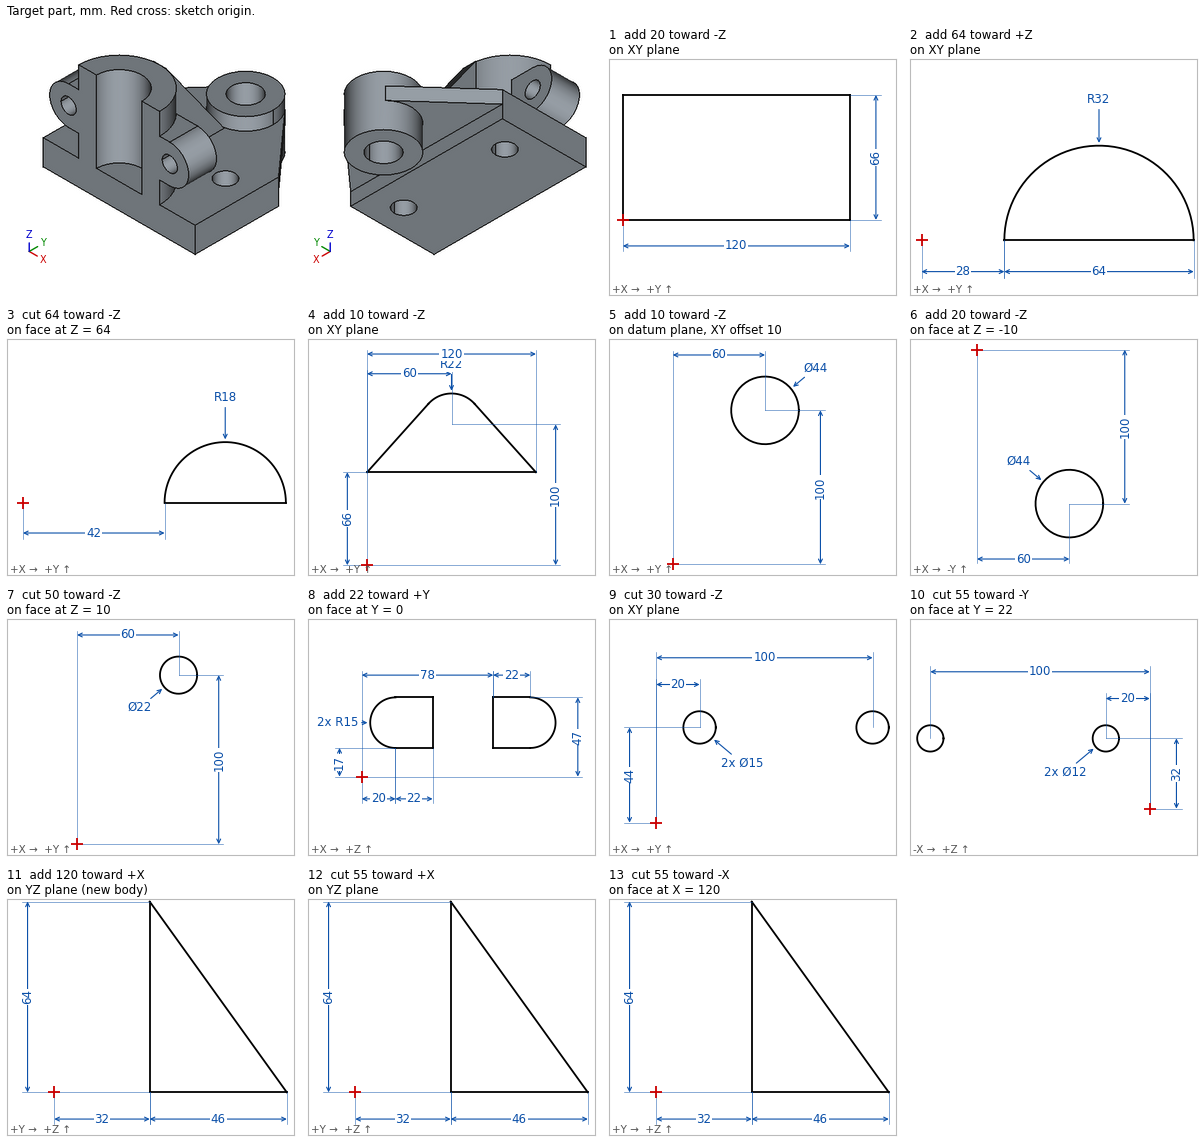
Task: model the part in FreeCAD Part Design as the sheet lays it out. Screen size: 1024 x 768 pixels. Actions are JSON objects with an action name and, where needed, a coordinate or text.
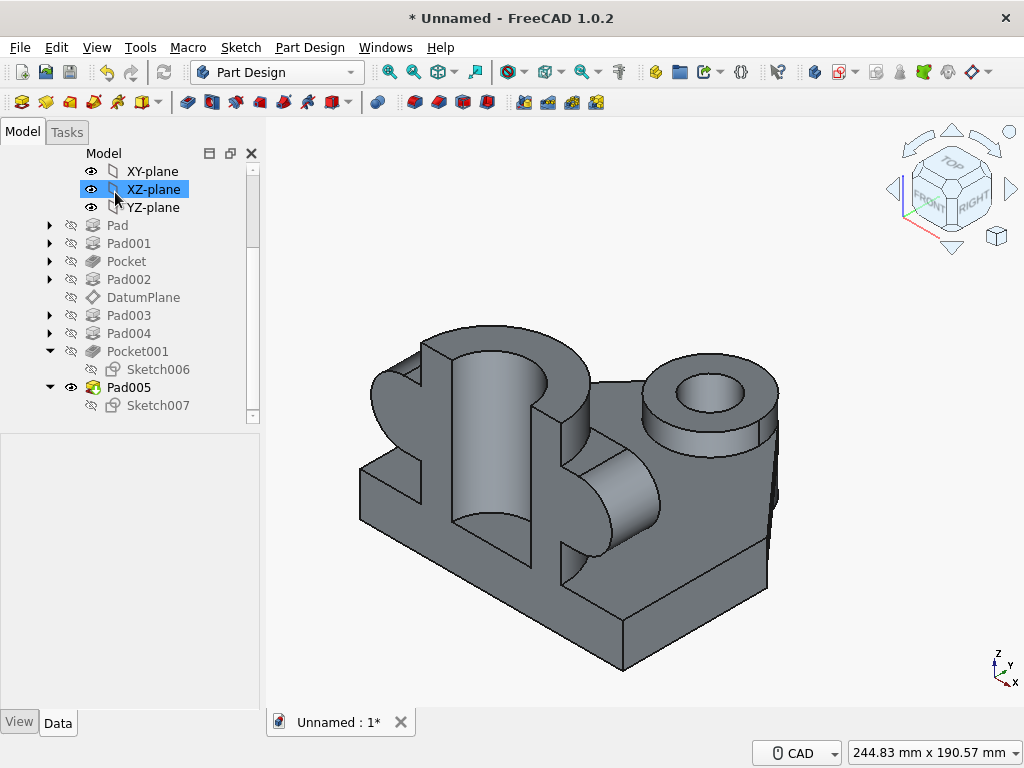
{"action": "left_click", "coordinate": [840, 72]}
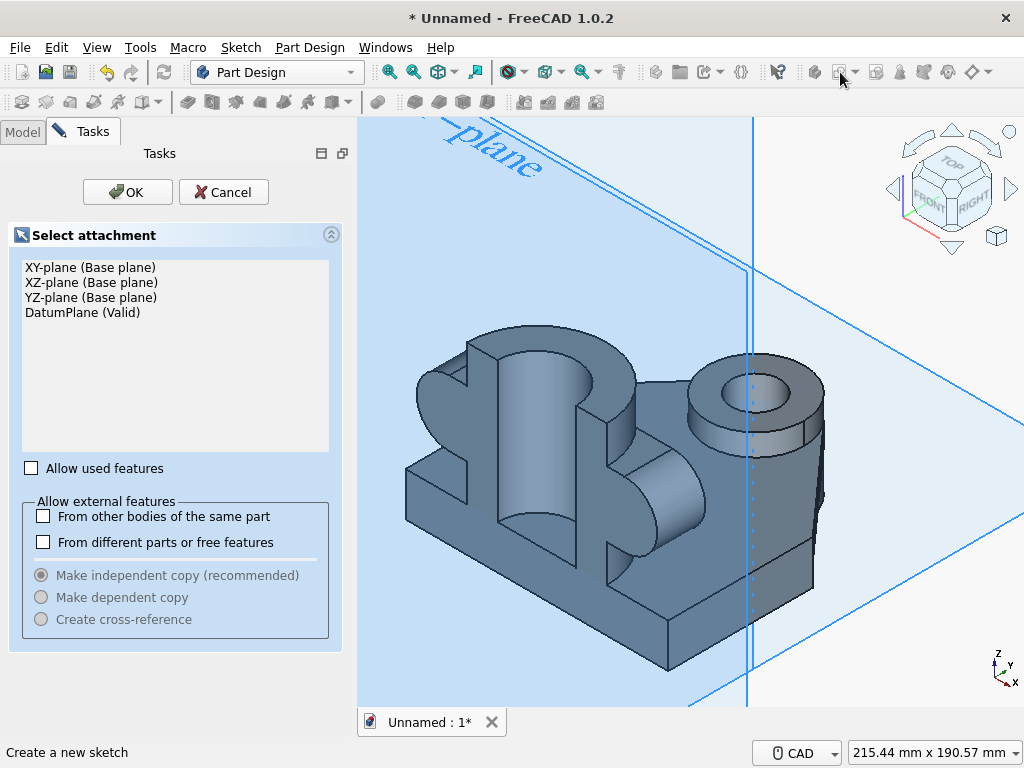
{"action": "left_click", "coordinate": [82, 268]}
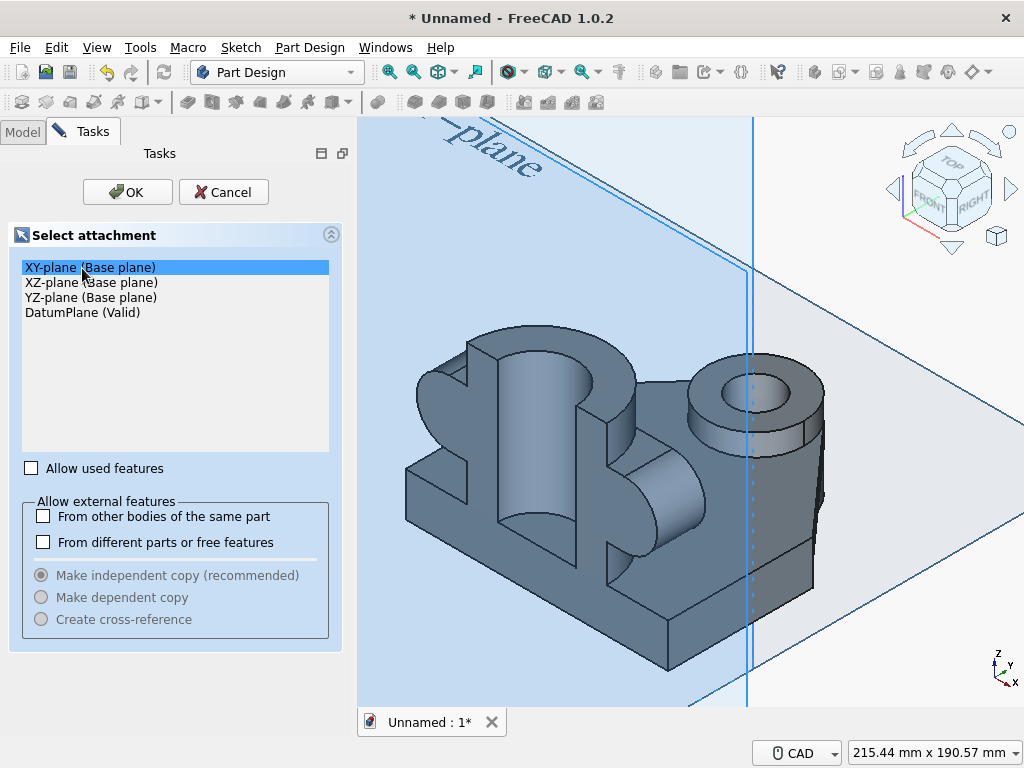
{"action": "left_click", "coordinate": [128, 192]}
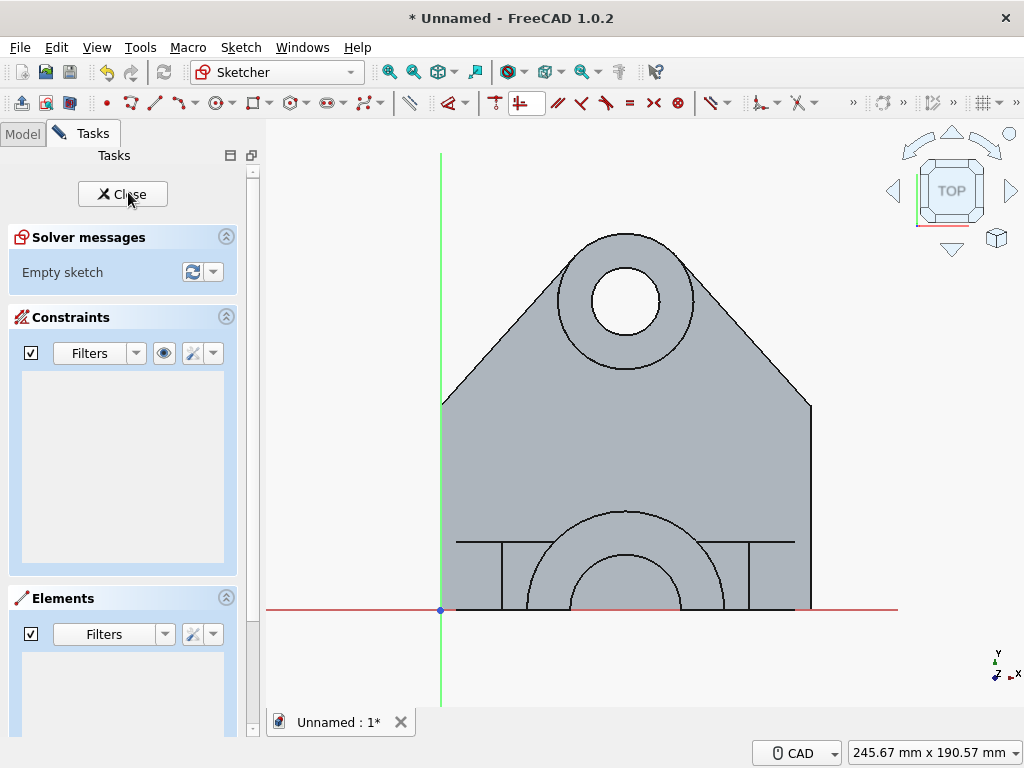
{"action": "left_click", "coordinate": [70, 104]}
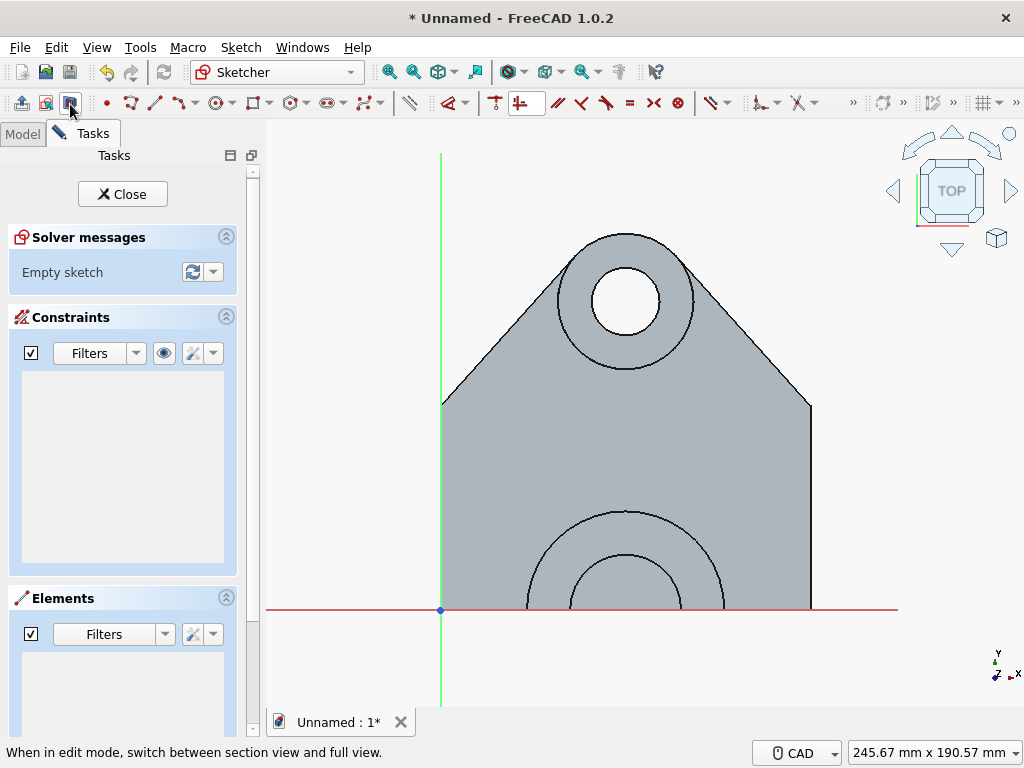
{"action": "left_click", "coordinate": [216, 104]}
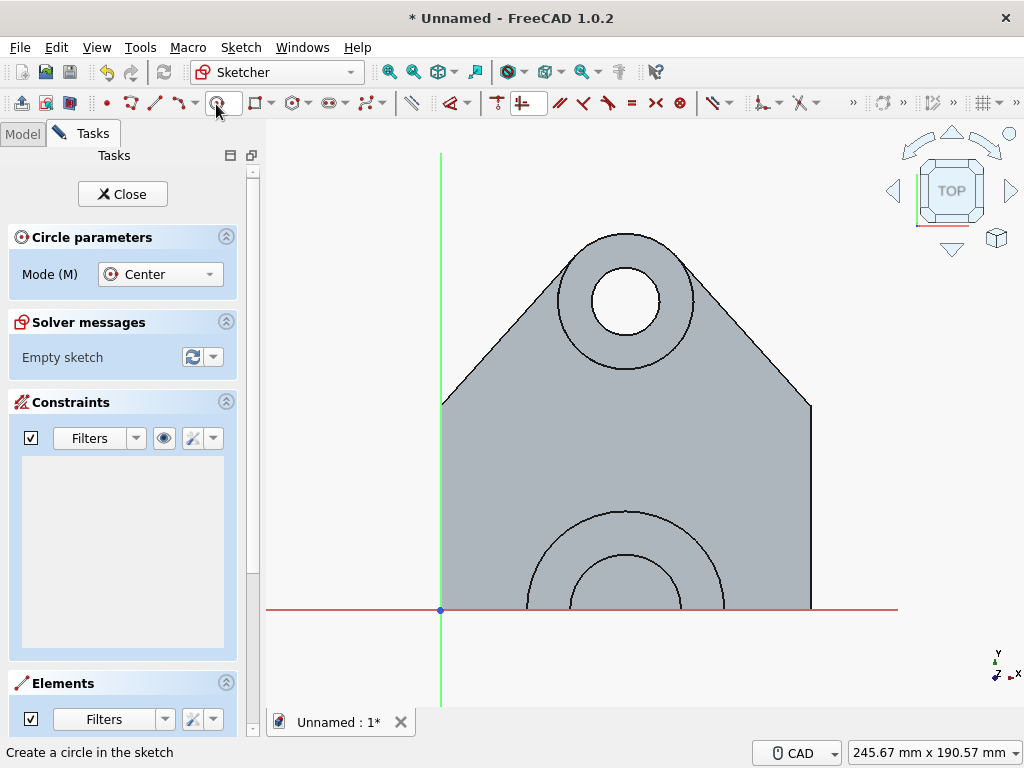
{"action": "left_click", "coordinate": [502, 474]}
{"action": "left_click", "coordinate": [519, 458]}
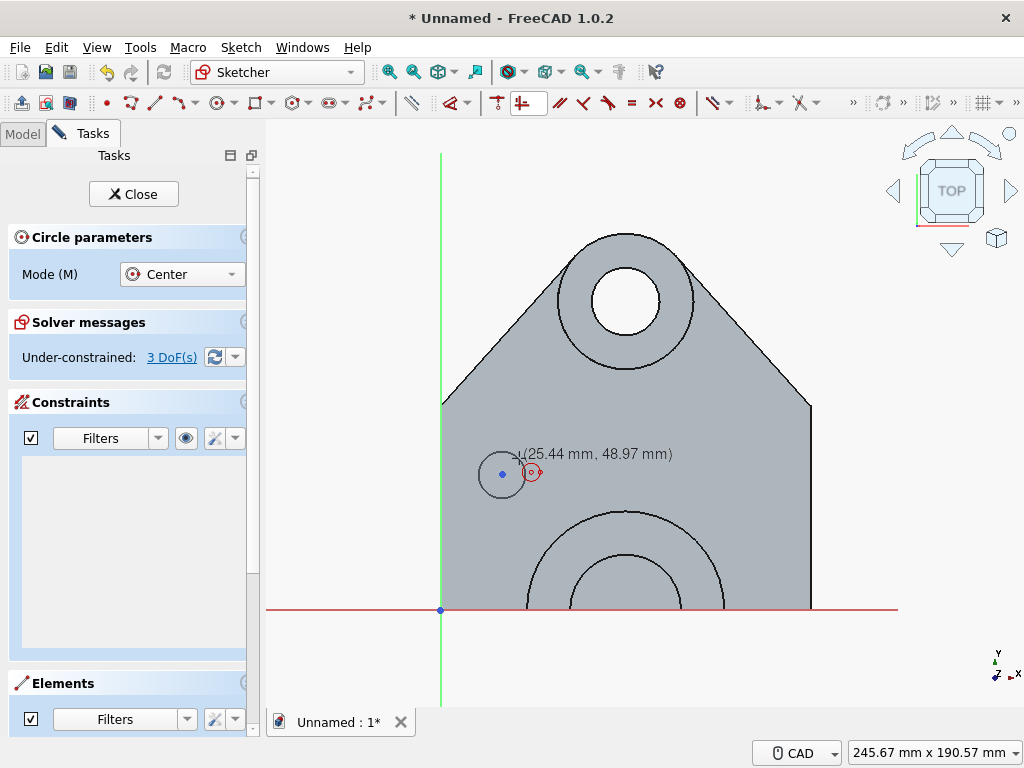
{"action": "left_click", "coordinate": [749, 474]}
{"action": "left_click", "coordinate": [765, 458]}
{"action": "key", "text": "Escape"}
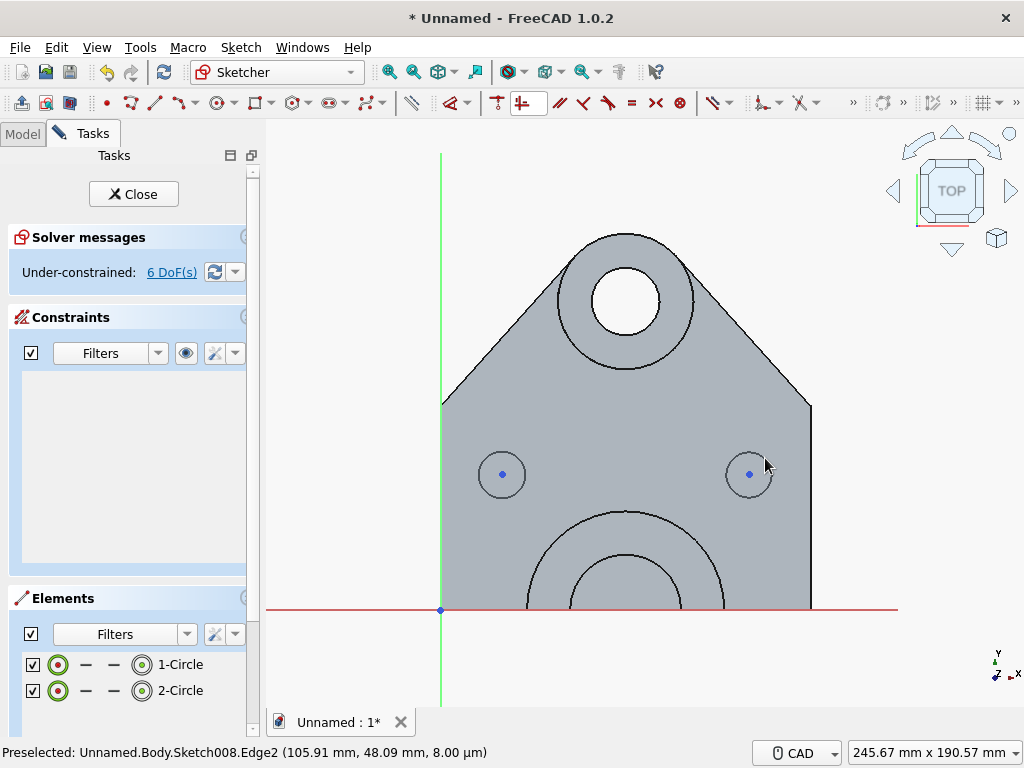
{"action": "left_click", "coordinate": [518, 458]}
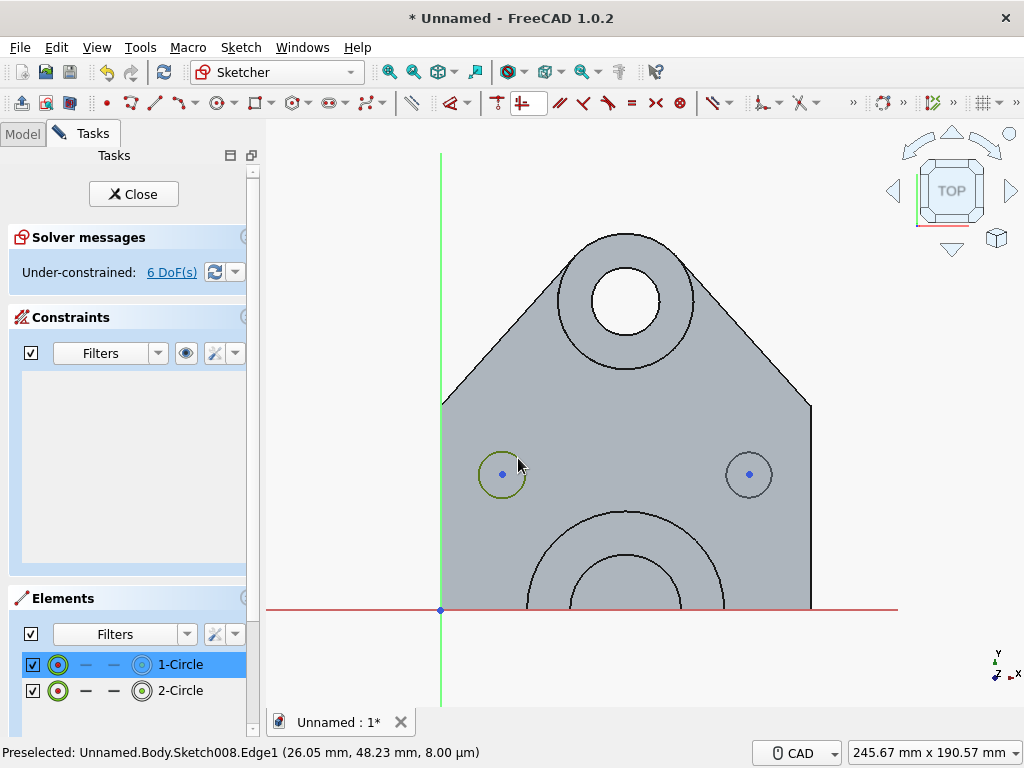
{"action": "left_click", "coordinate": [765, 459]}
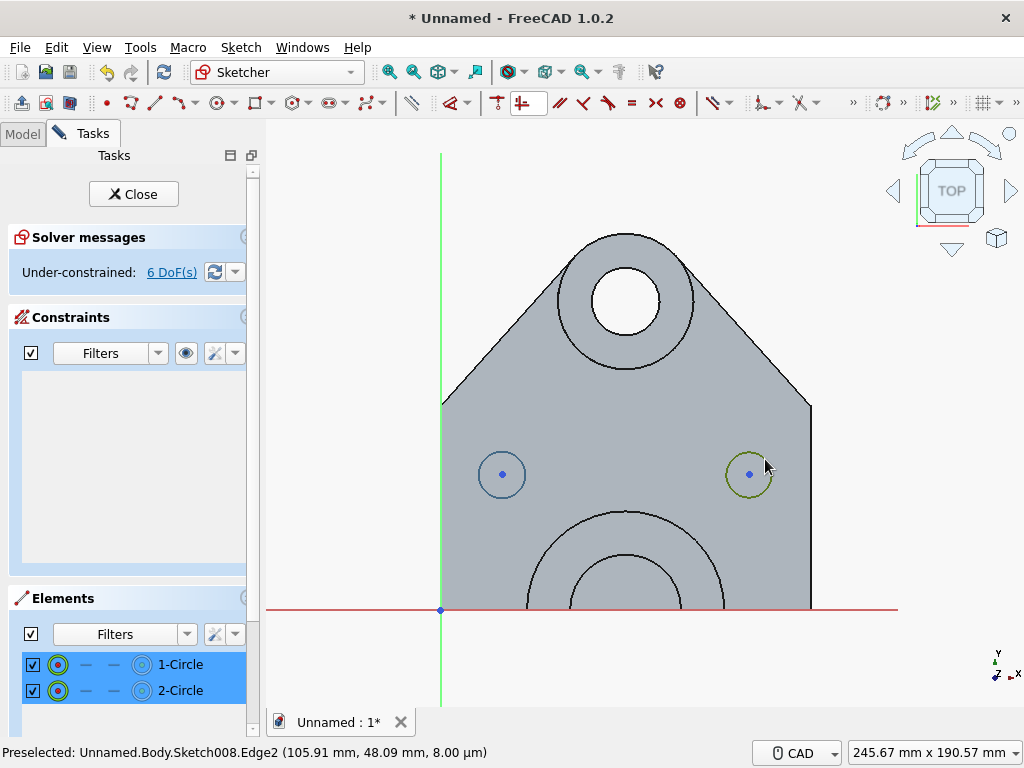
{"action": "left_click", "coordinate": [632, 104]}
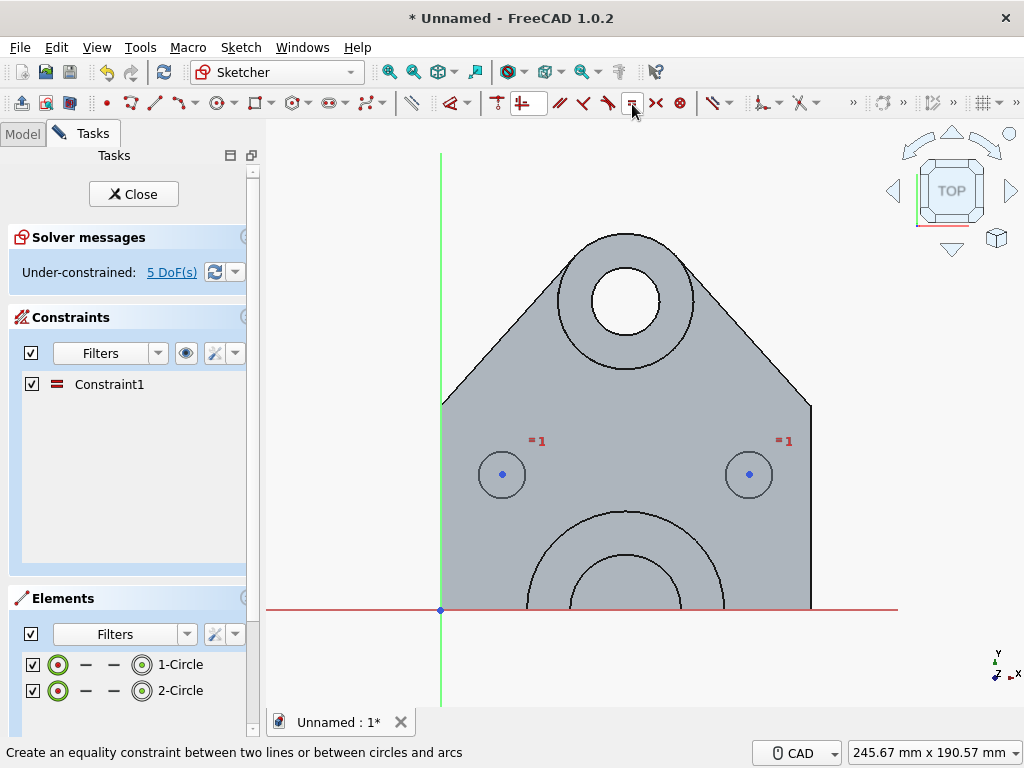
{"action": "left_click", "coordinate": [502, 475]}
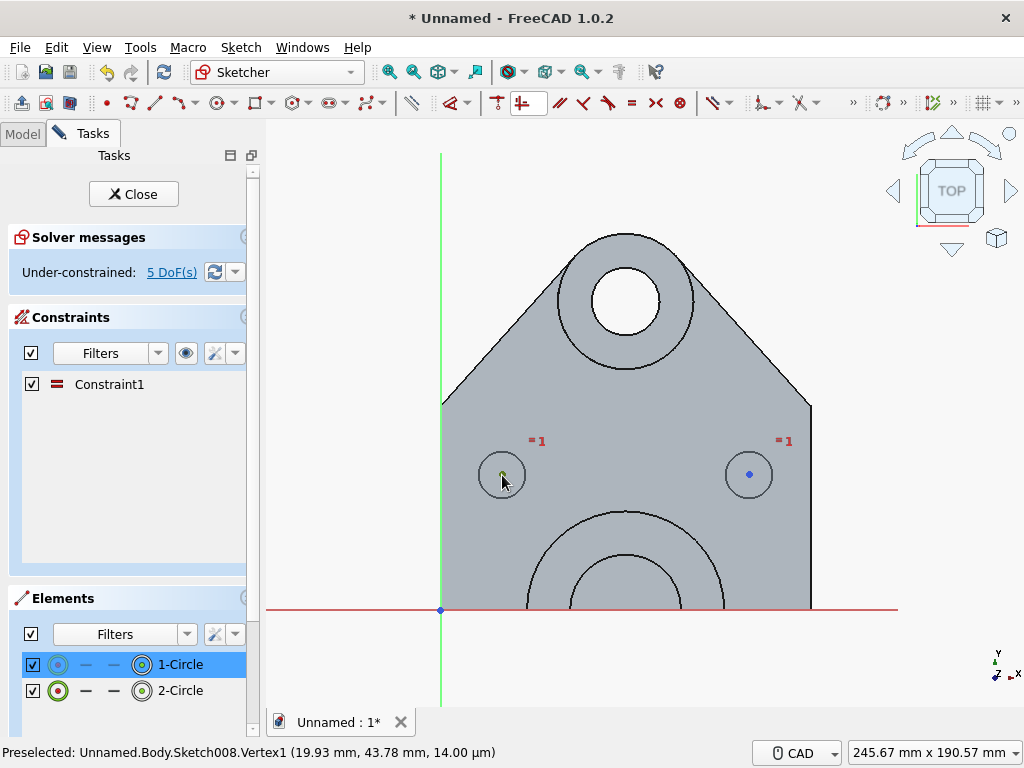
{"action": "left_click", "coordinate": [749, 475]}